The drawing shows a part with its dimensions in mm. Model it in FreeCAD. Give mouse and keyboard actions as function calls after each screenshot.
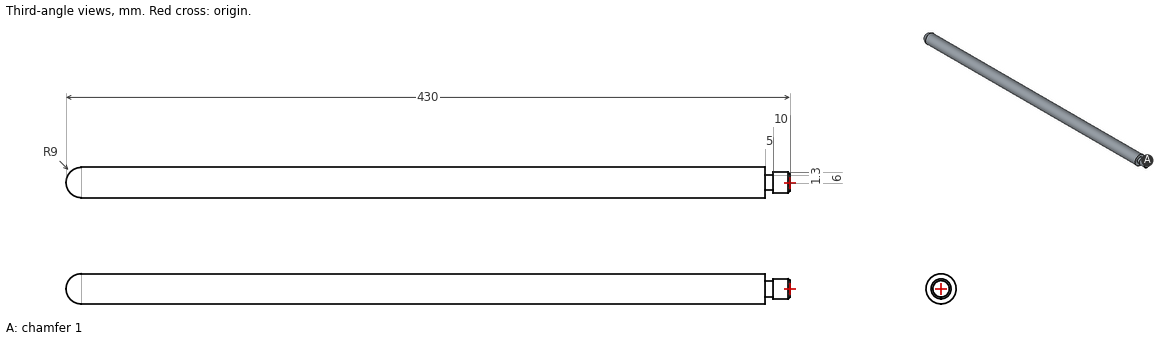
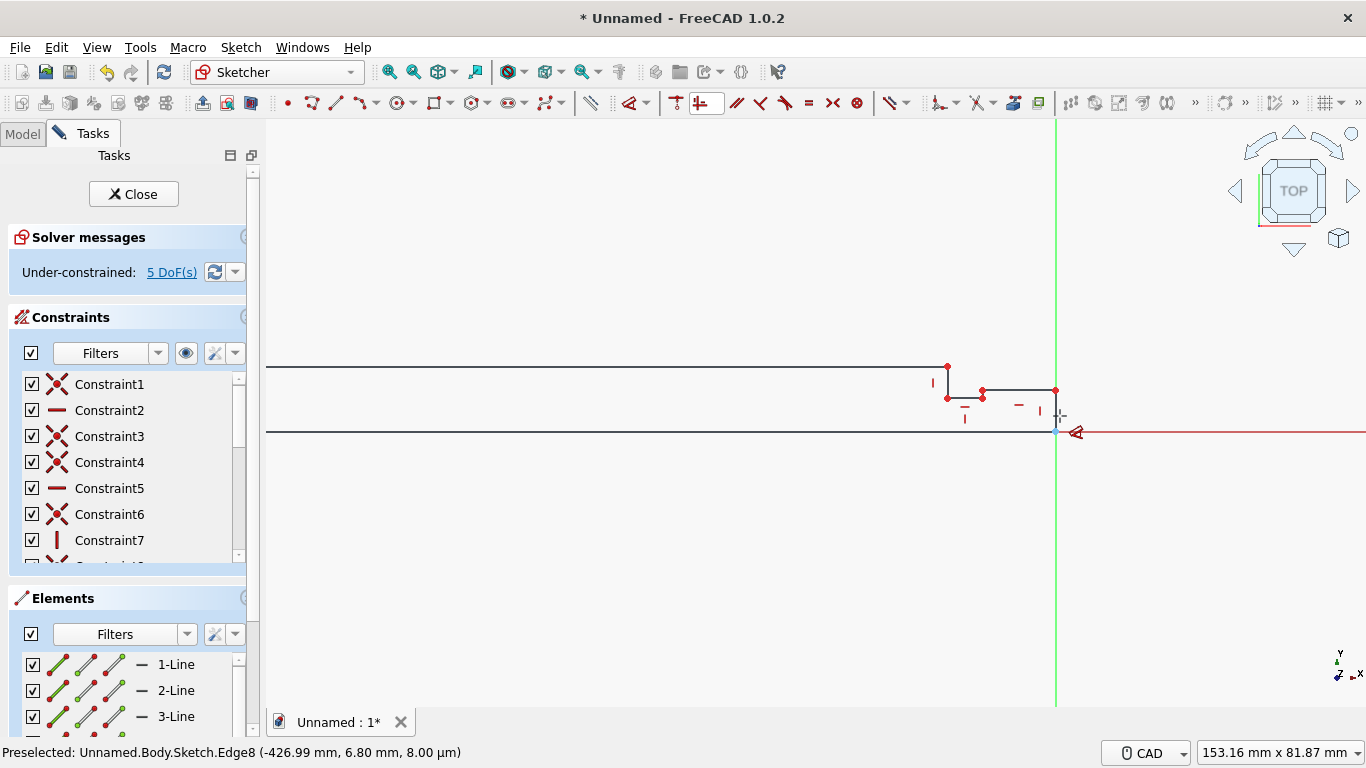
click(1056, 415)
click(1090, 411)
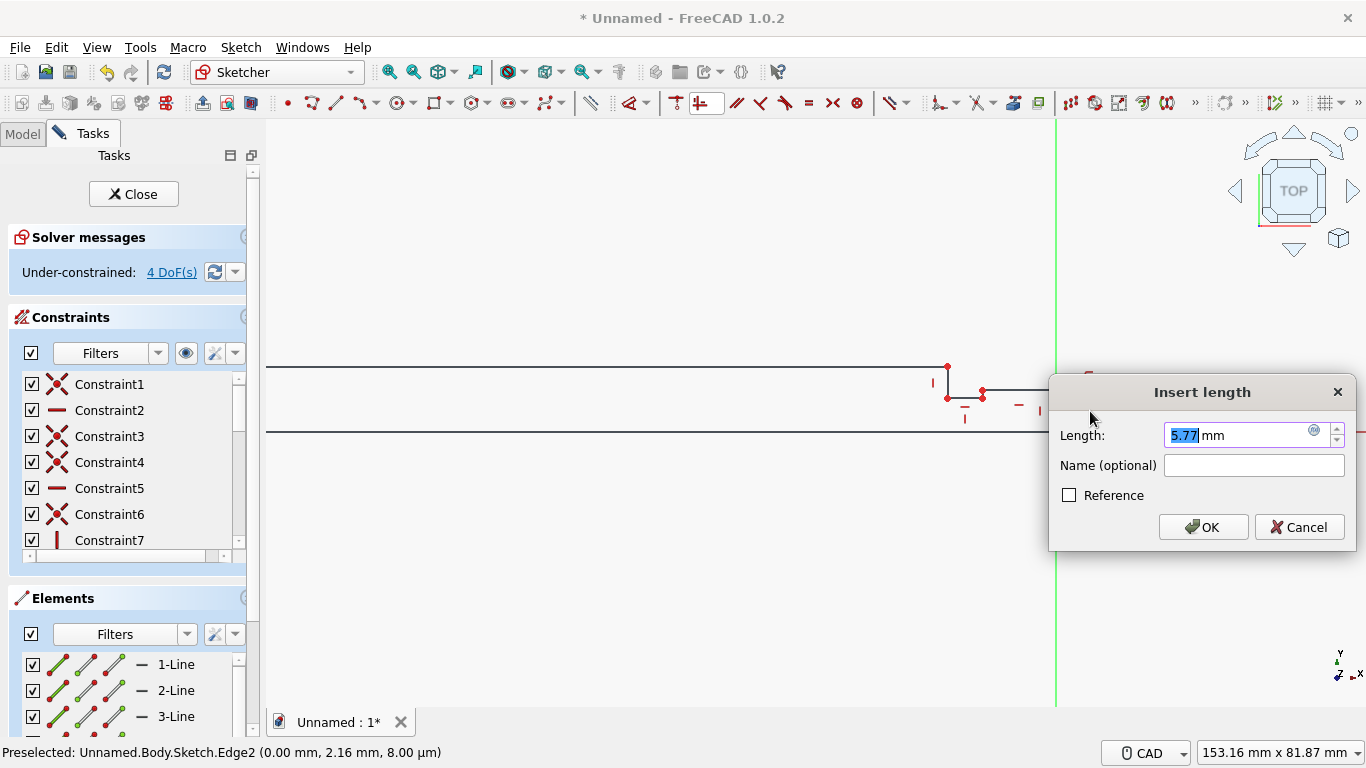
text(6)
key(Return)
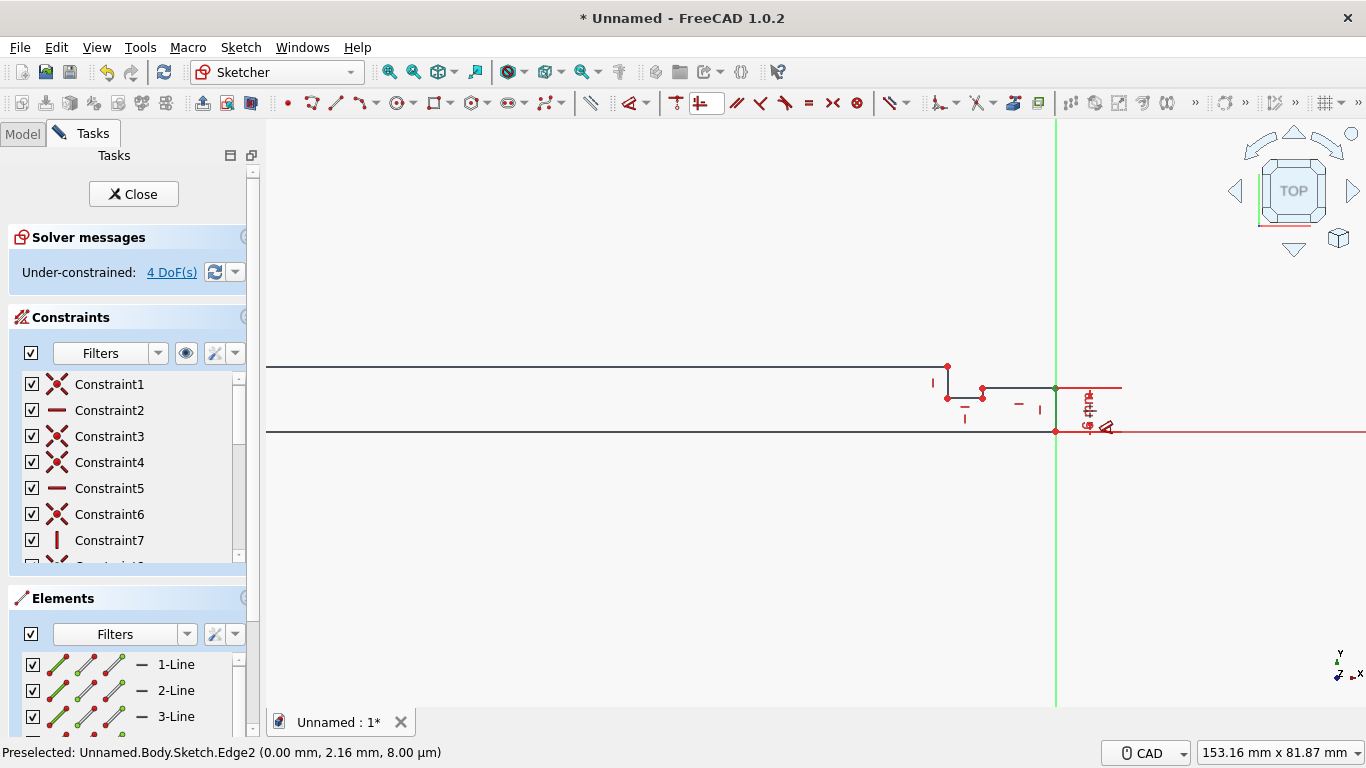
scroll(972, 398, up, 2)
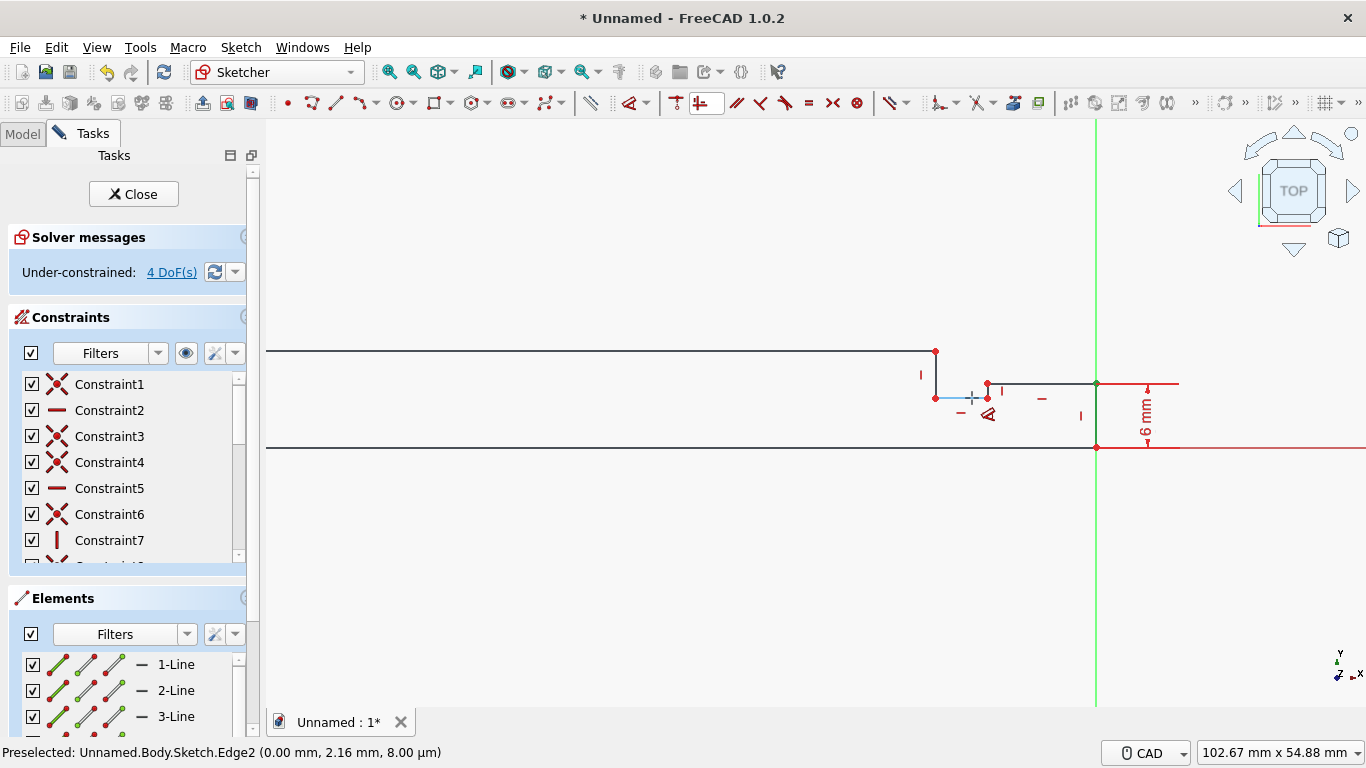
click(972, 398)
click(962, 364)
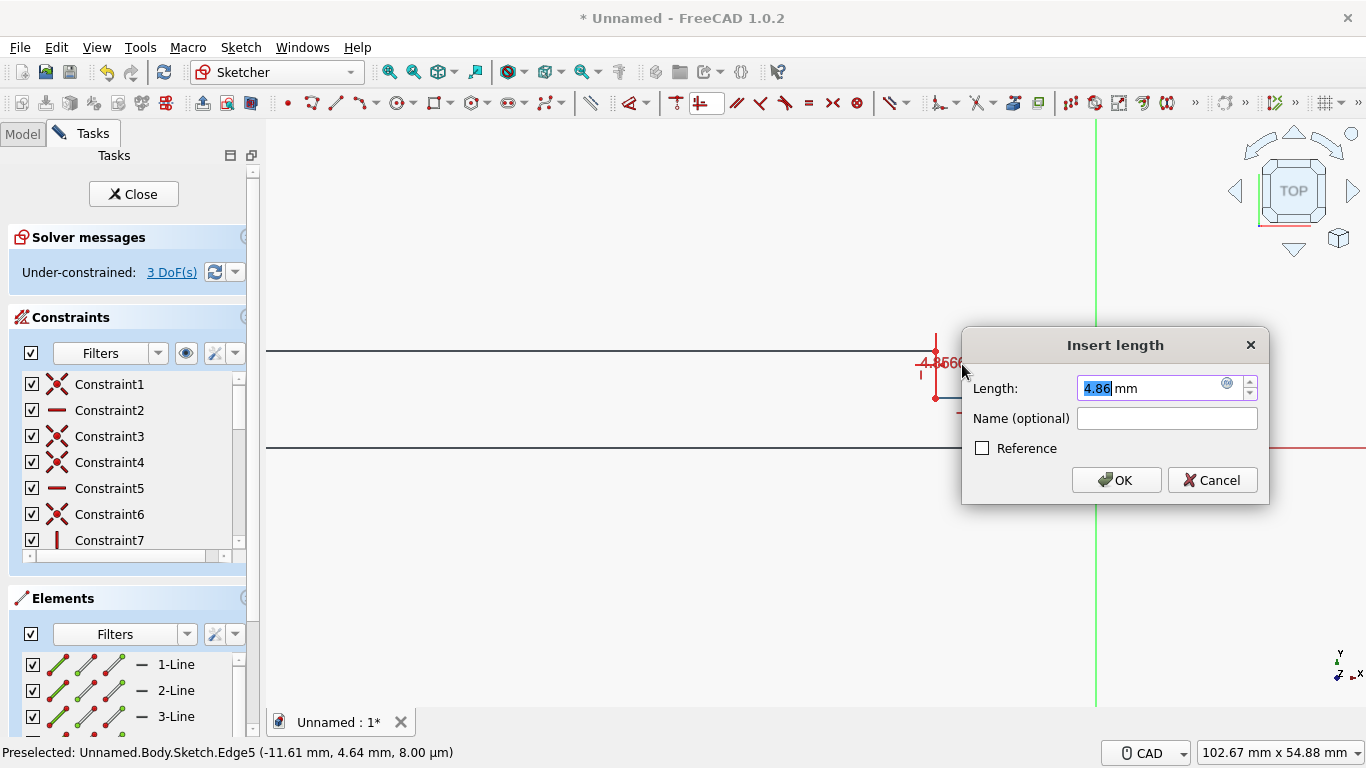
text(5)
key(Return)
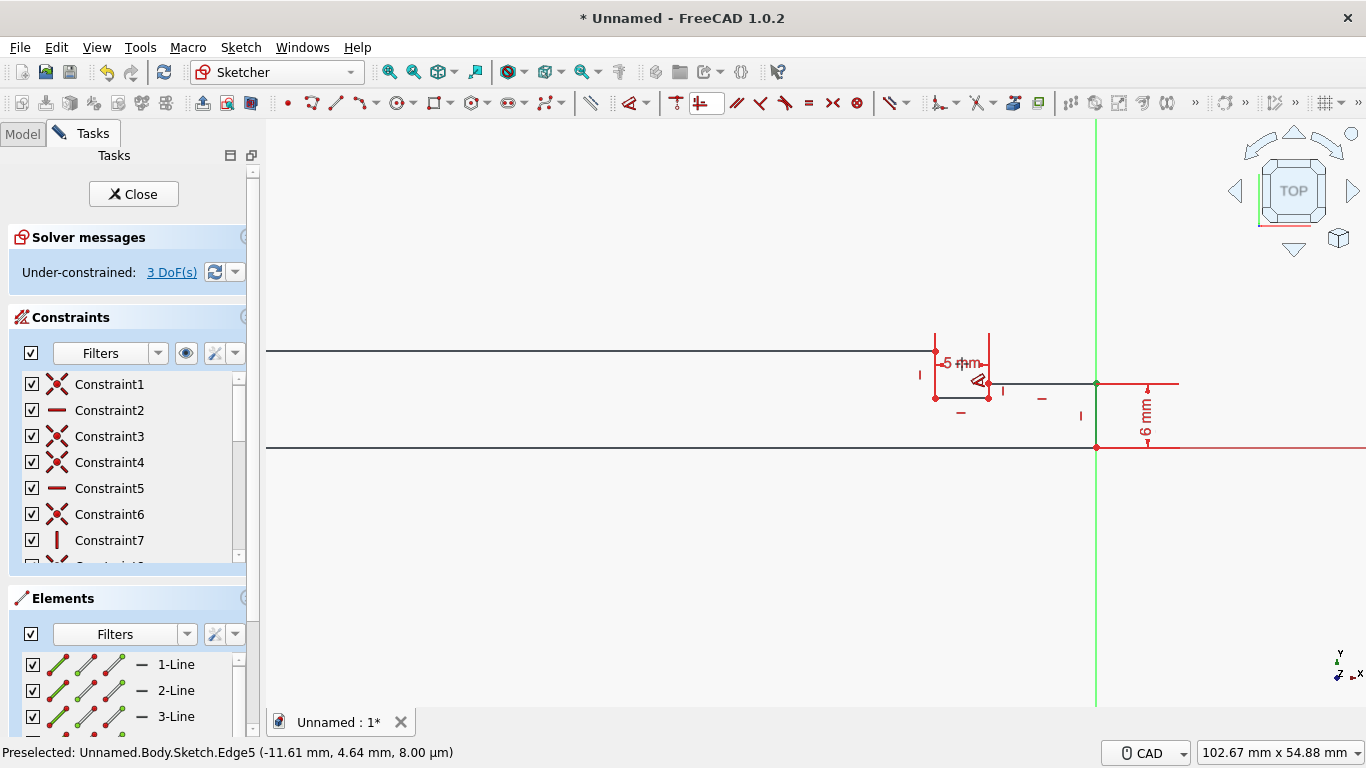
click(1064, 384)
click(1043, 350)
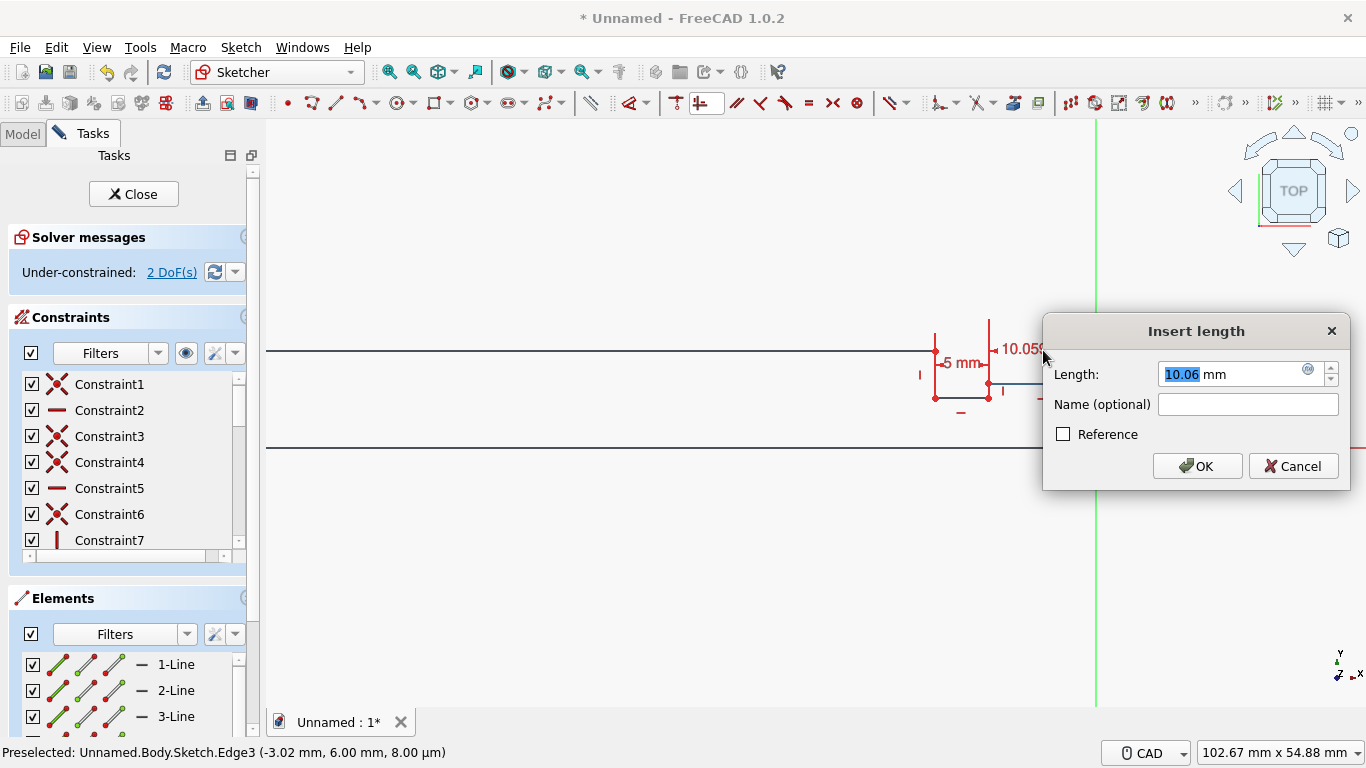
text(10)
key(Return)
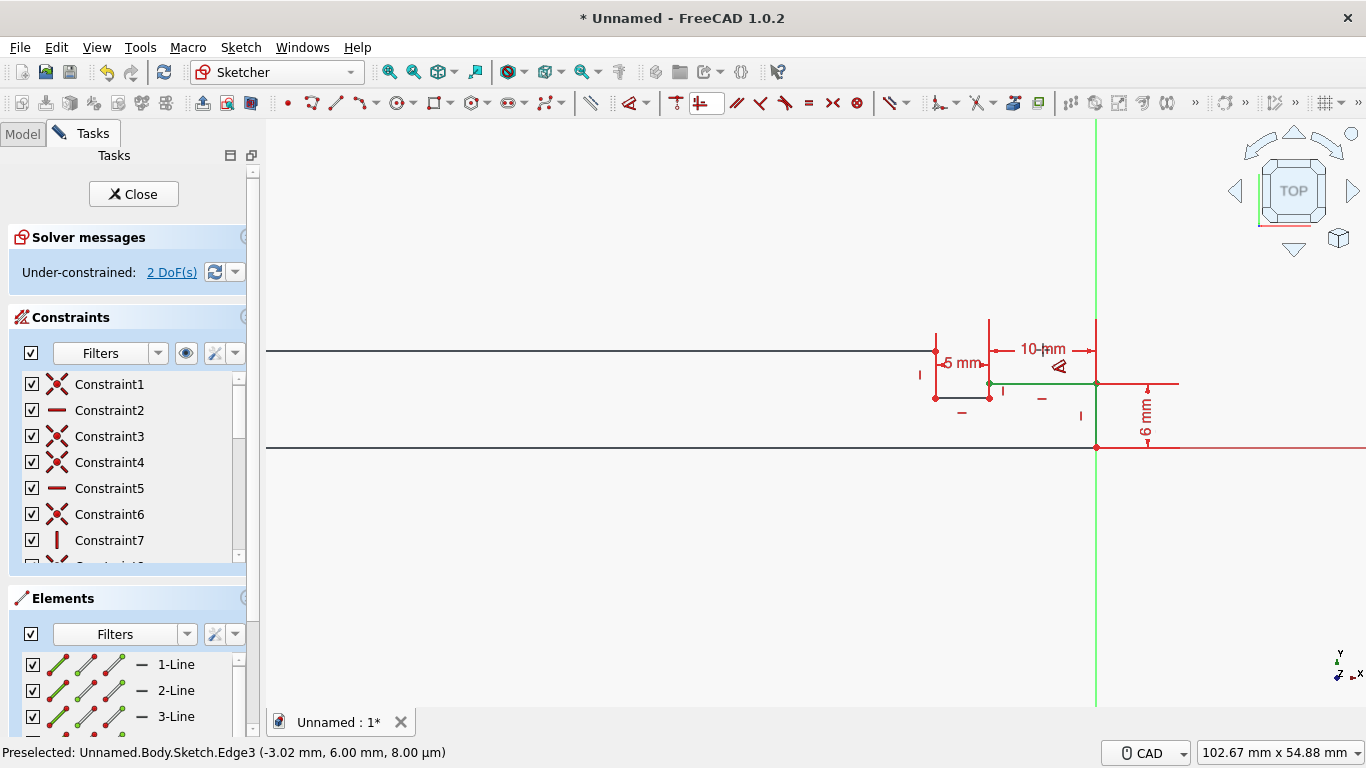
scroll(1053, 415, down, 10)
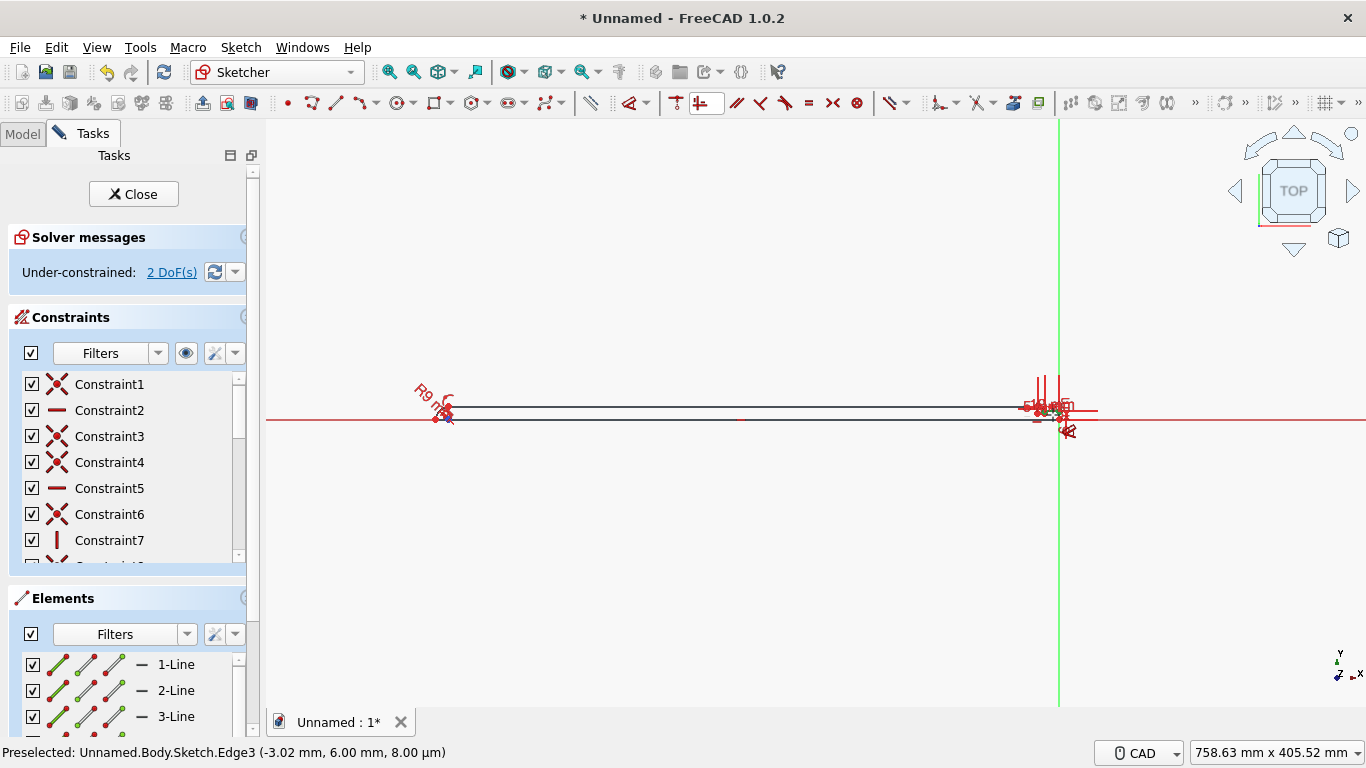
click(623, 420)
click(748, 454)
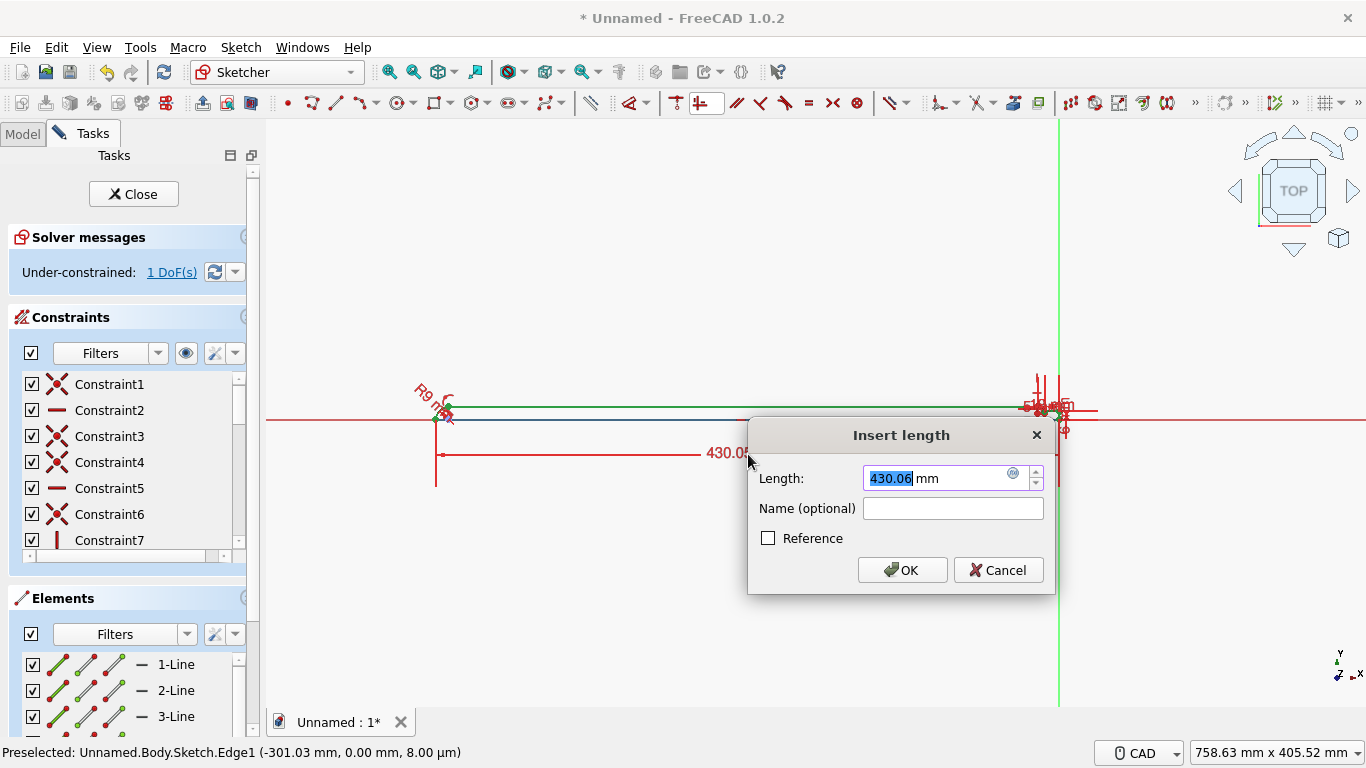
text(430)
key(Return)